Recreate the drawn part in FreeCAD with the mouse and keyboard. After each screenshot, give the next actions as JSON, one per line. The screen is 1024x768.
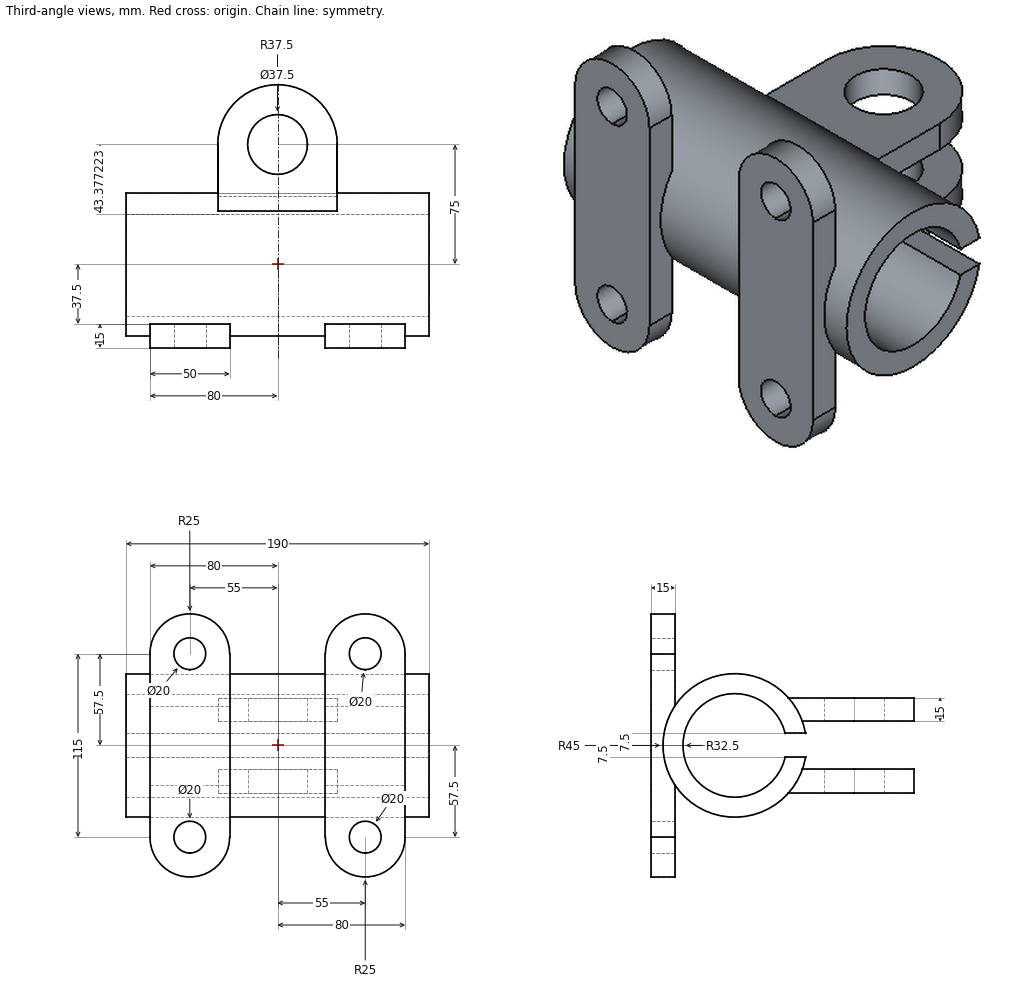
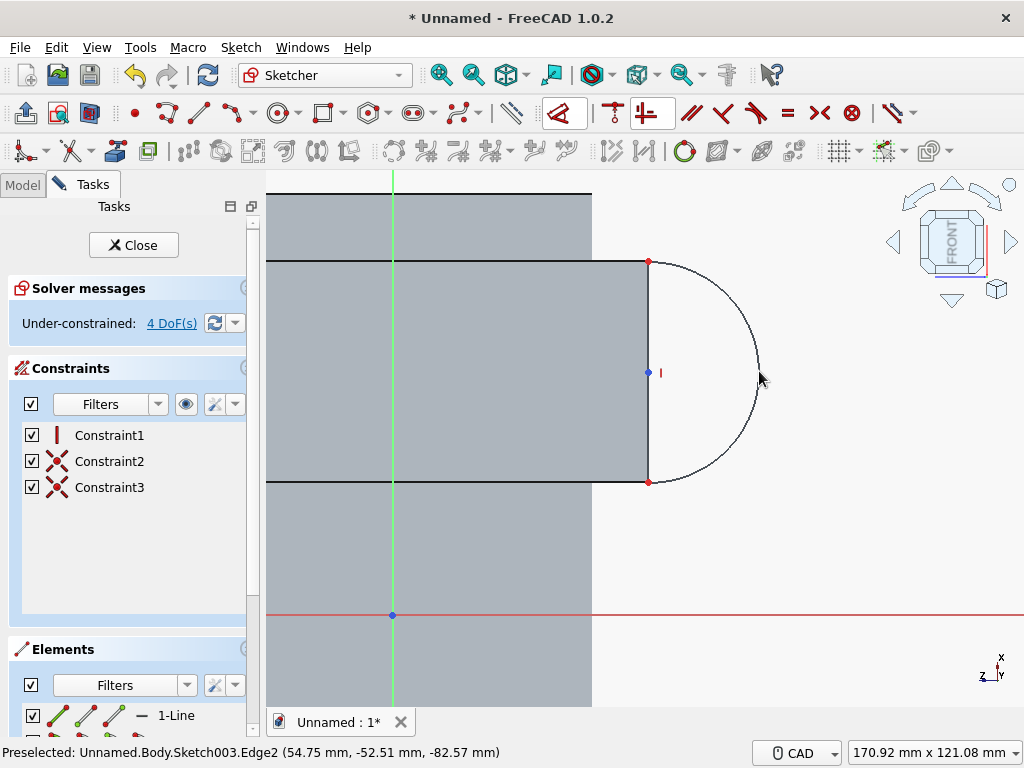
{"action": "left_click", "coordinate": [738, 438]}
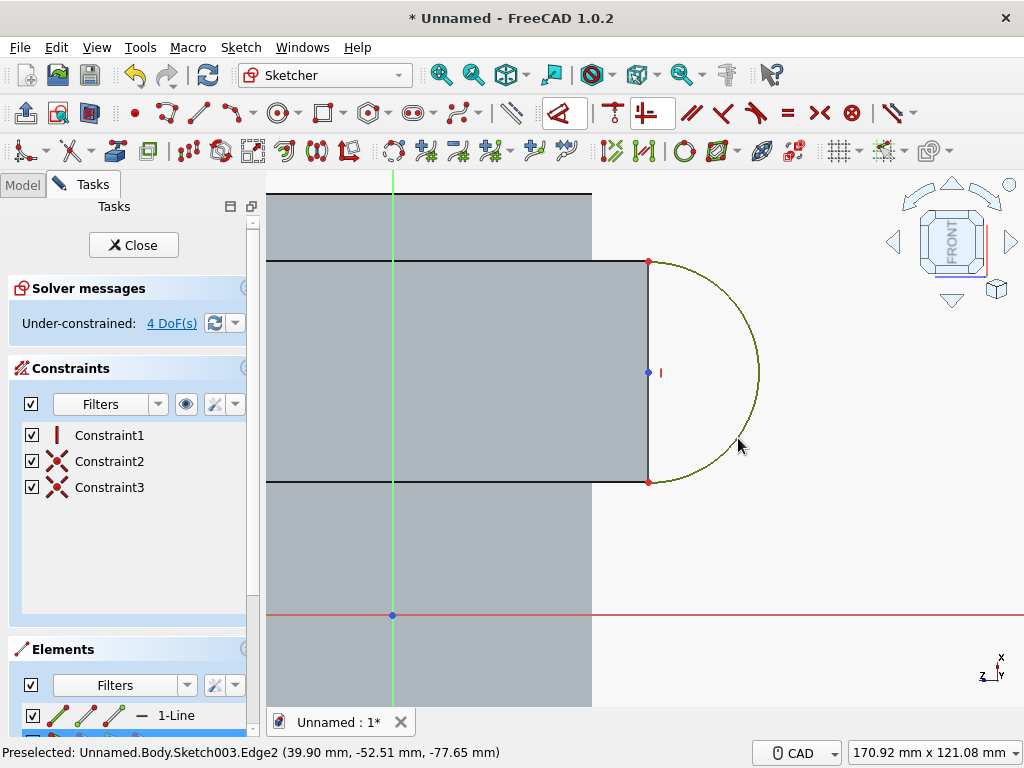
{"action": "left_click", "coordinate": [582, 114]}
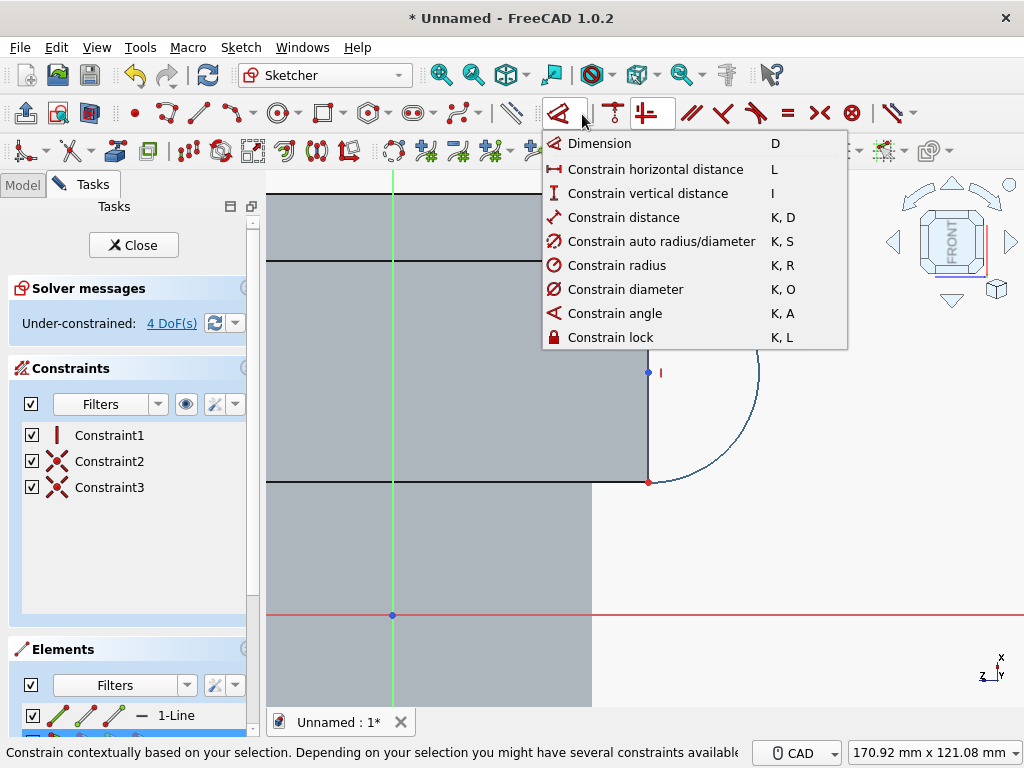
{"action": "left_click", "coordinate": [695, 265]}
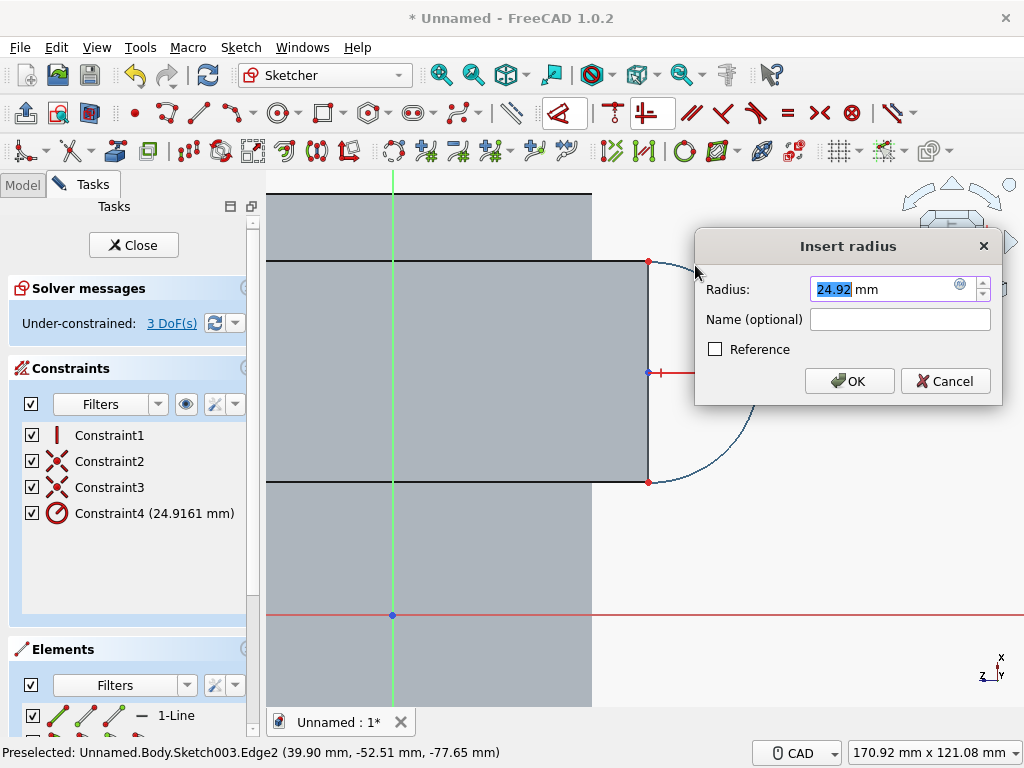
{"action": "type", "text": "25"}
{"action": "key", "text": "Return"}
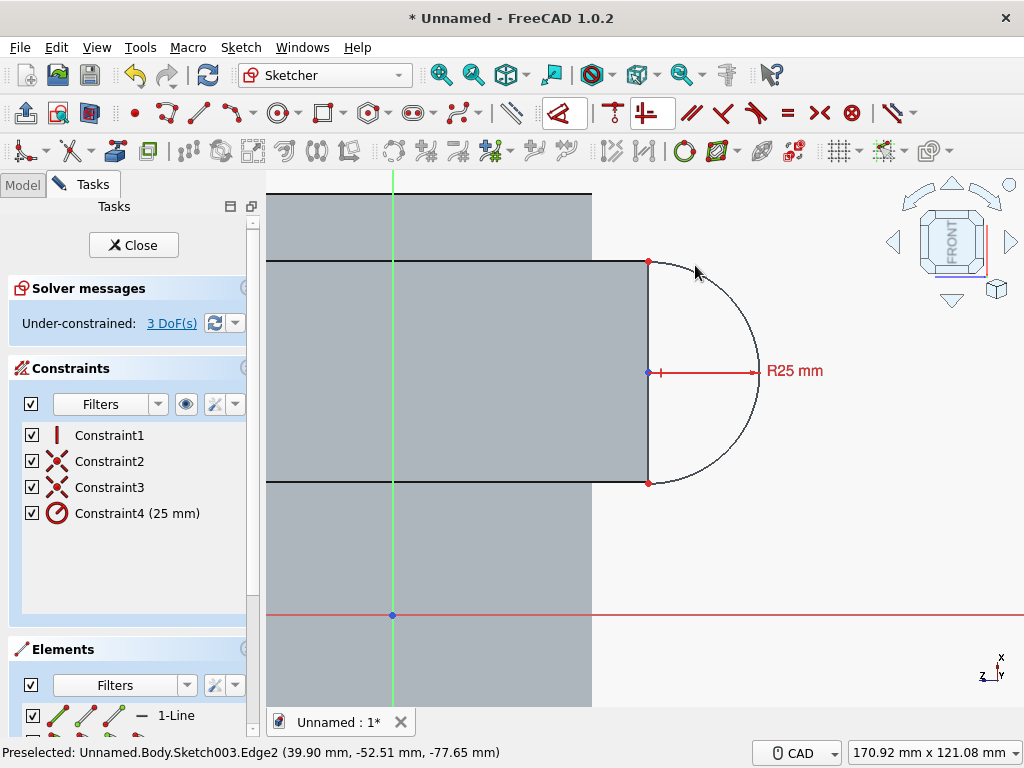
{"action": "left_click", "coordinate": [648, 262]}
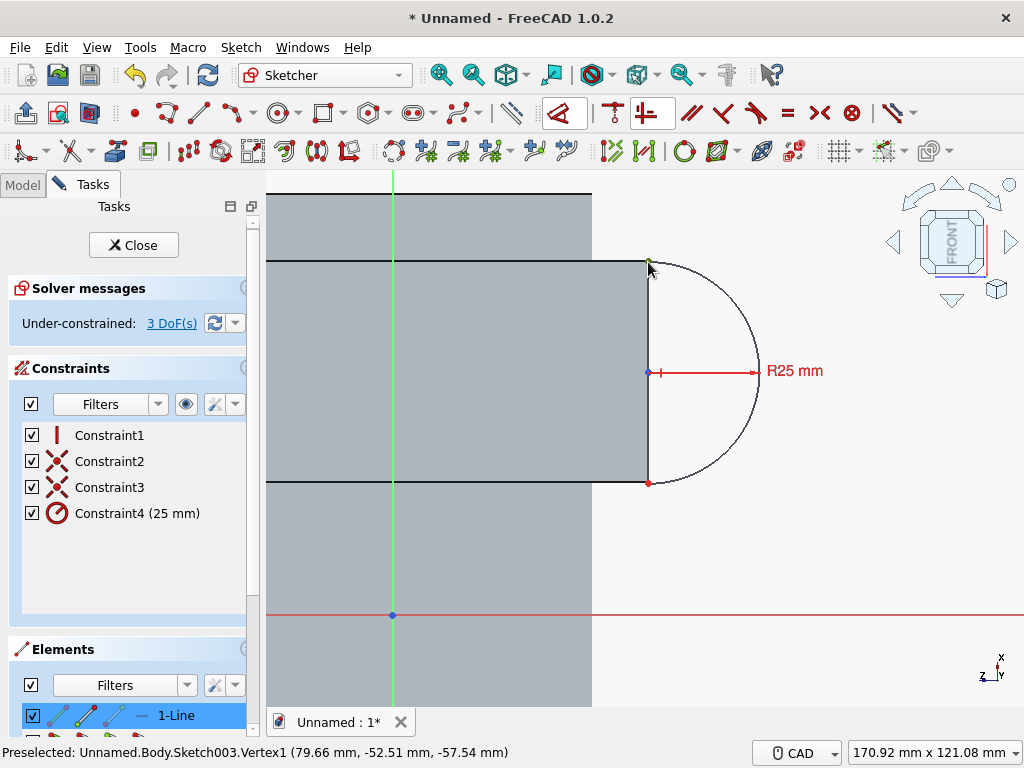
{"action": "left_click", "coordinate": [582, 114]}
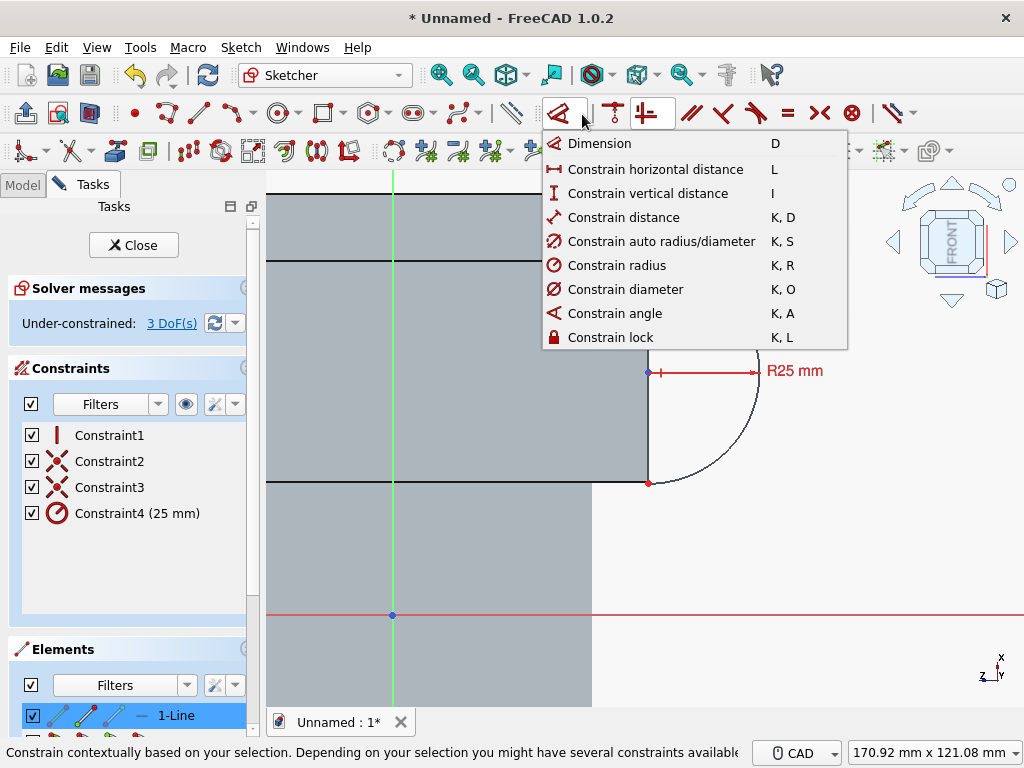
{"action": "left_click", "coordinate": [695, 193]}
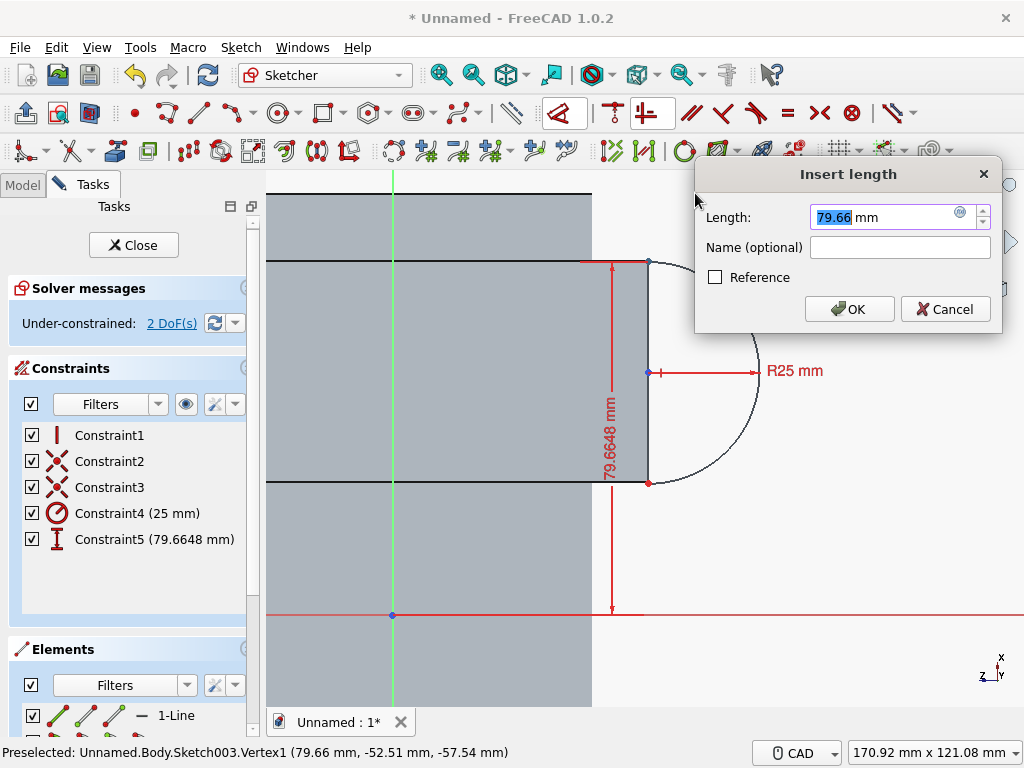
{"action": "type", "text": "80"}
{"action": "key", "text": "Return"}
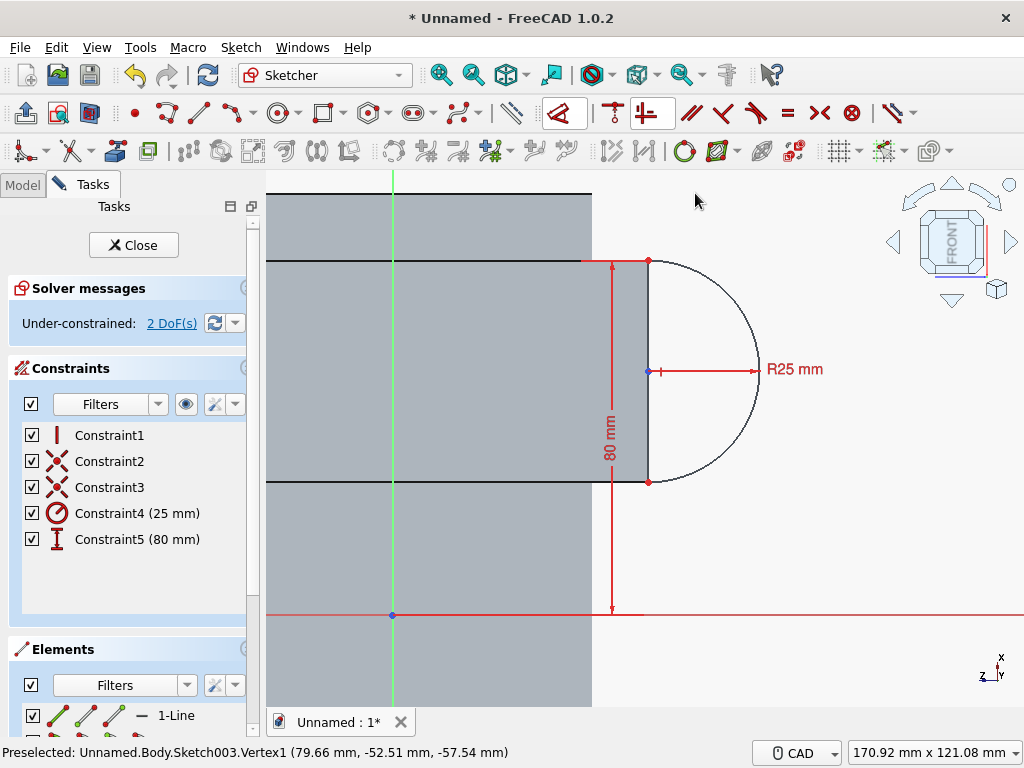
{"action": "left_click", "coordinate": [648, 261]}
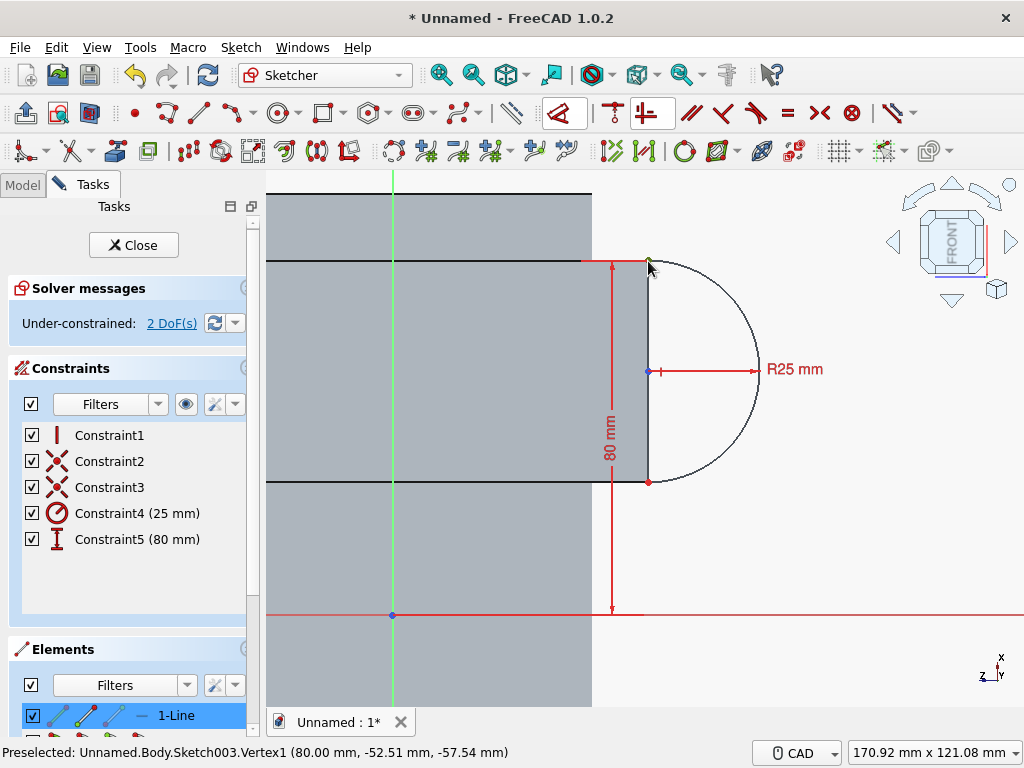
{"action": "left_click", "coordinate": [582, 114]}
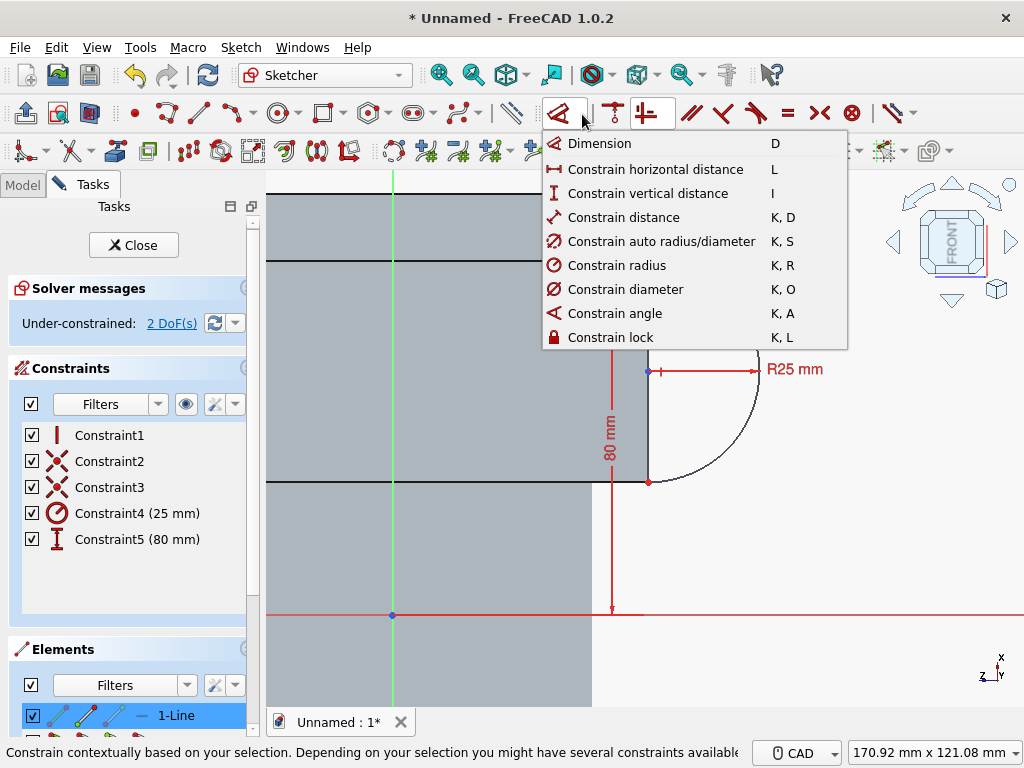
{"action": "left_click", "coordinate": [695, 169]}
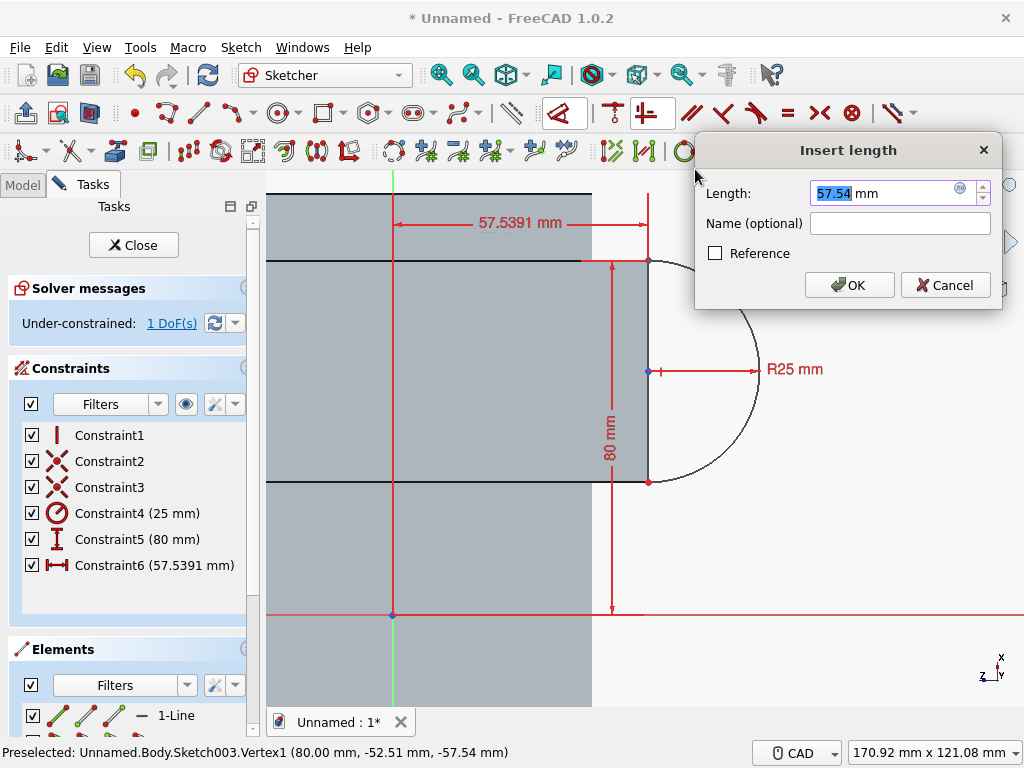
{"action": "type", "text": "57.5"}
{"action": "key", "text": "Return"}